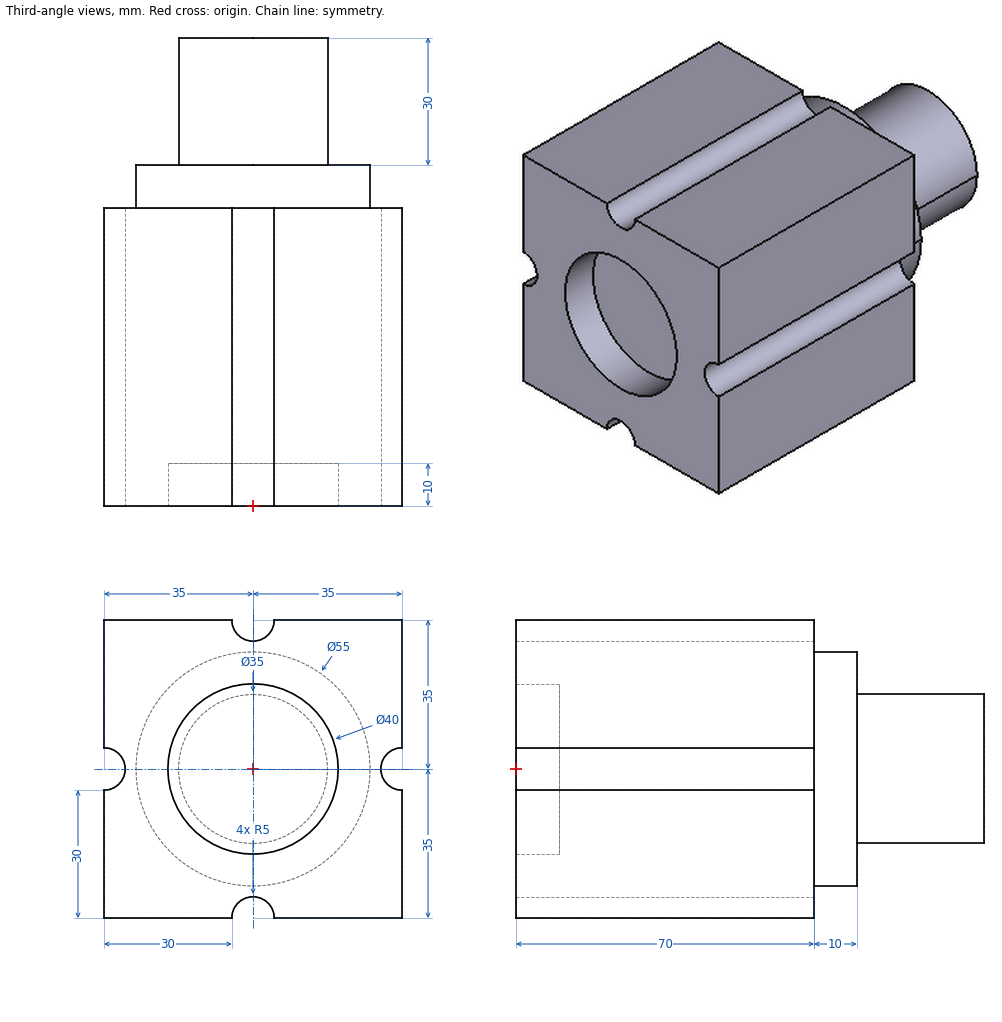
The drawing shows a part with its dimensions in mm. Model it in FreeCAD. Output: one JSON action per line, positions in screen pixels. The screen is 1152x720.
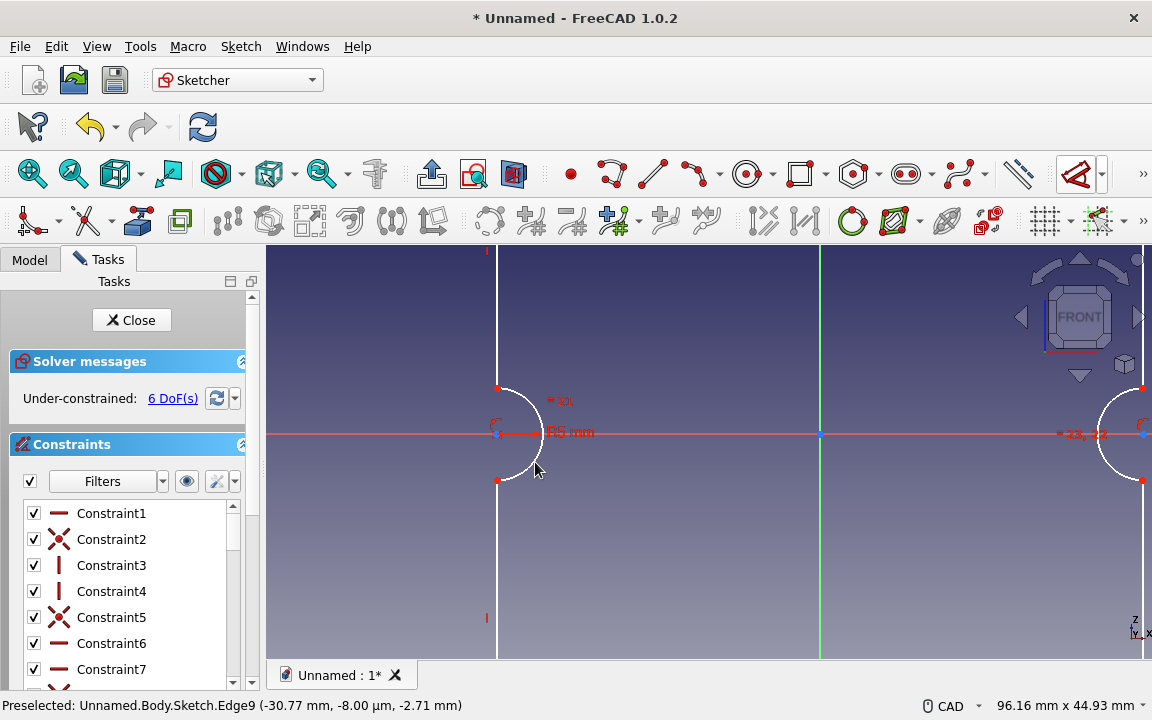
{"action": "scroll", "coordinate": [536, 462], "scroll_direction": "down", "scroll_amount": 5}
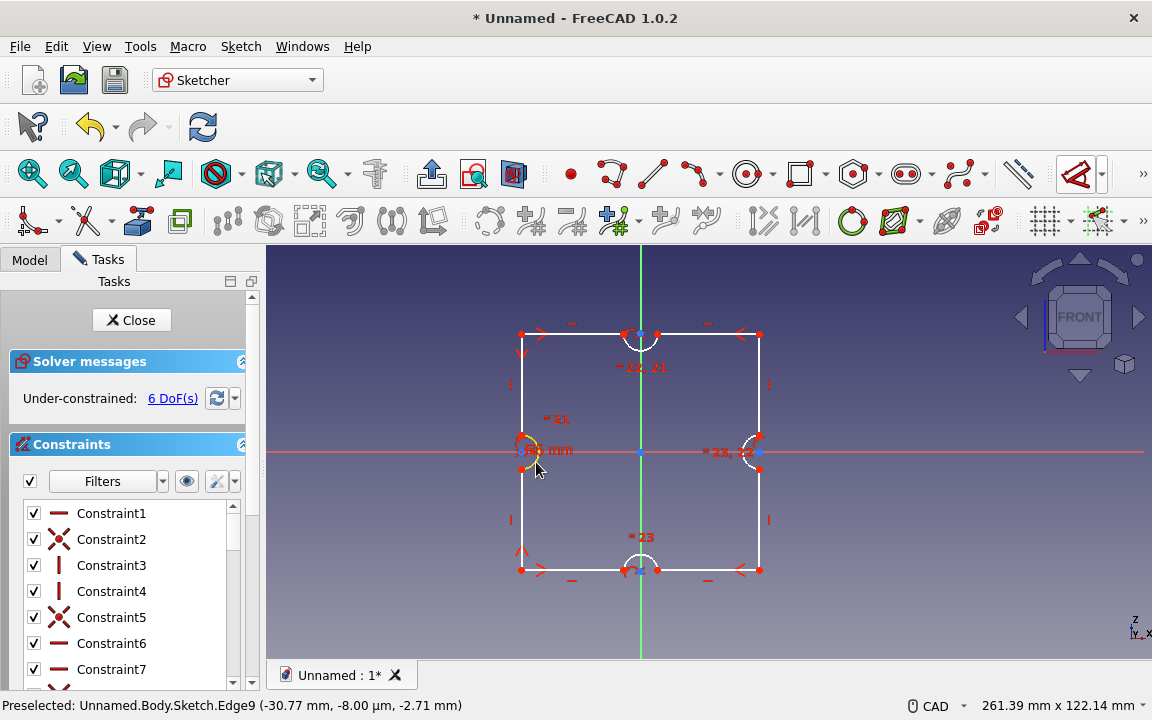
{"action": "left_click", "coordinate": [593, 570]}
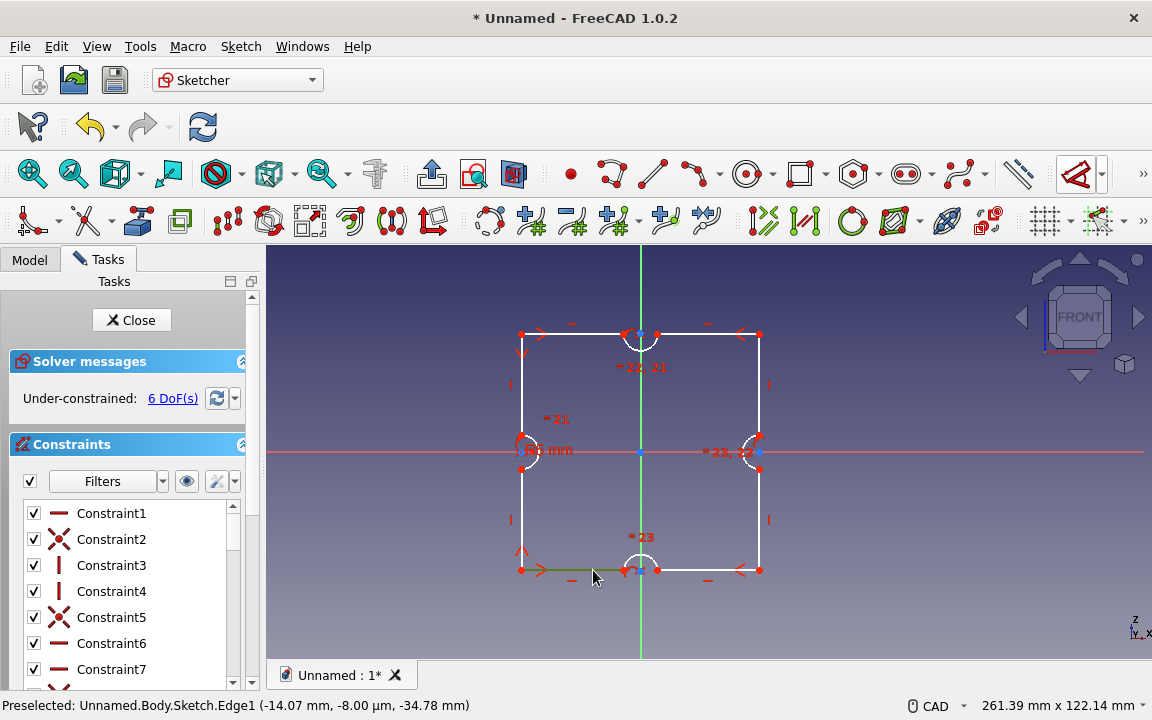
{"action": "key", "text": "l"}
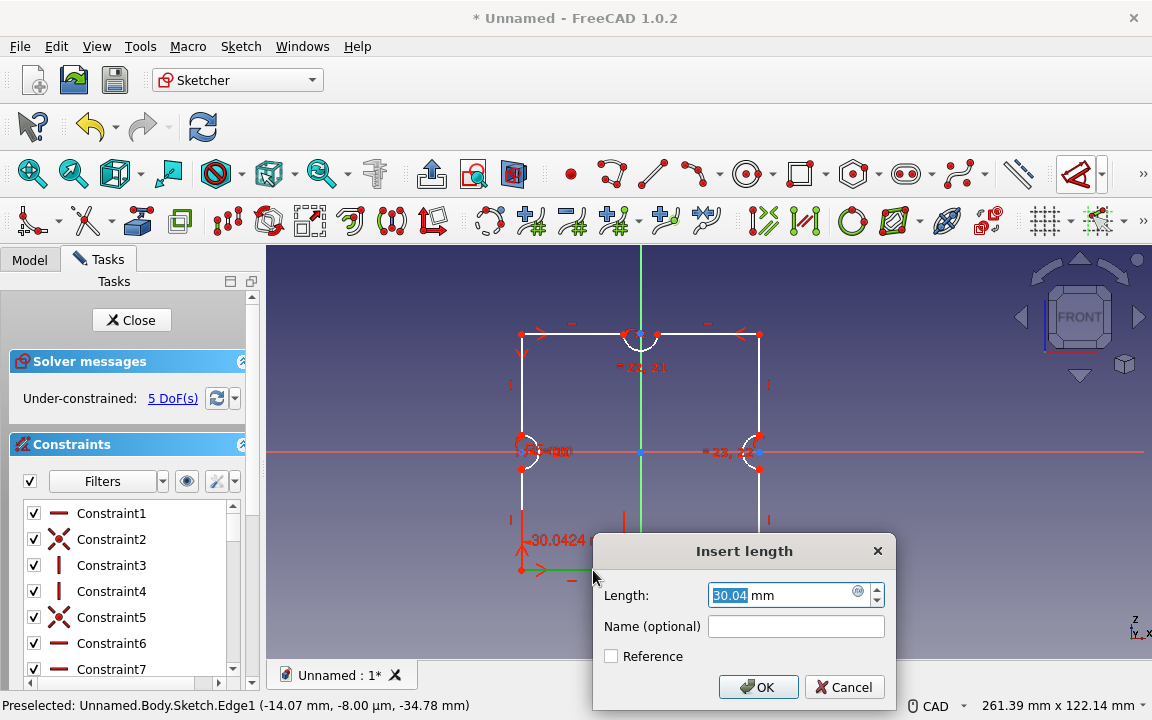
{"action": "type", "text": "30"}
{"action": "key", "text": "Return"}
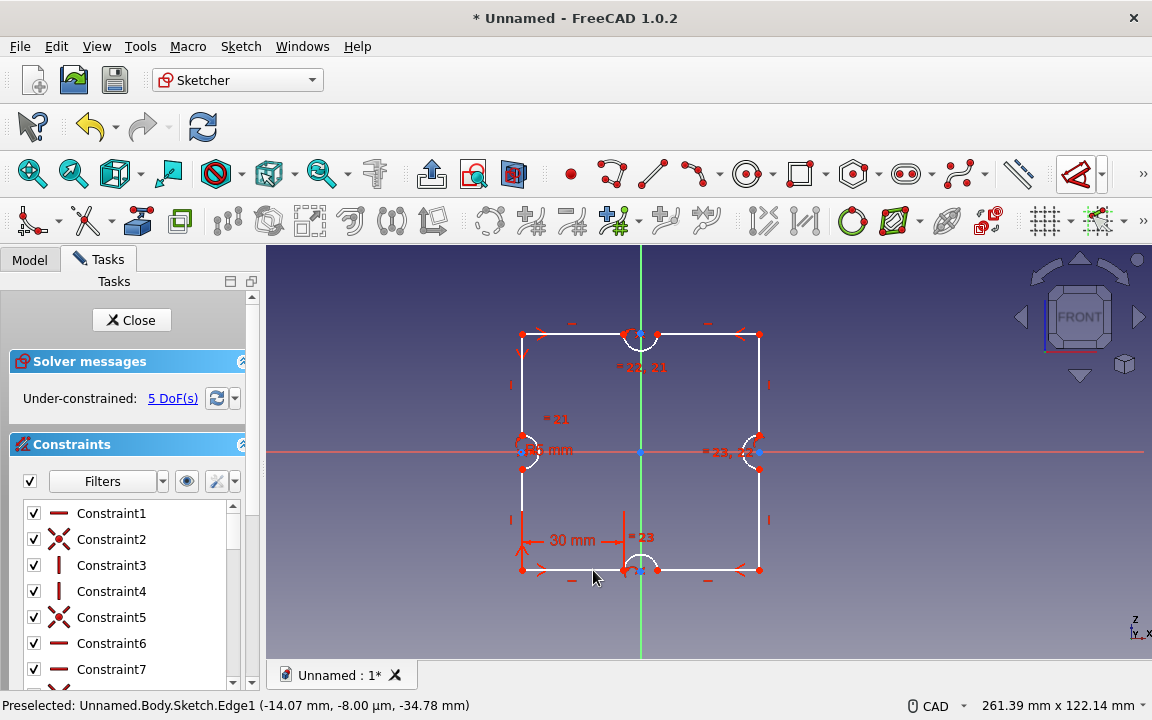
{"action": "left_click", "coordinate": [522, 499]}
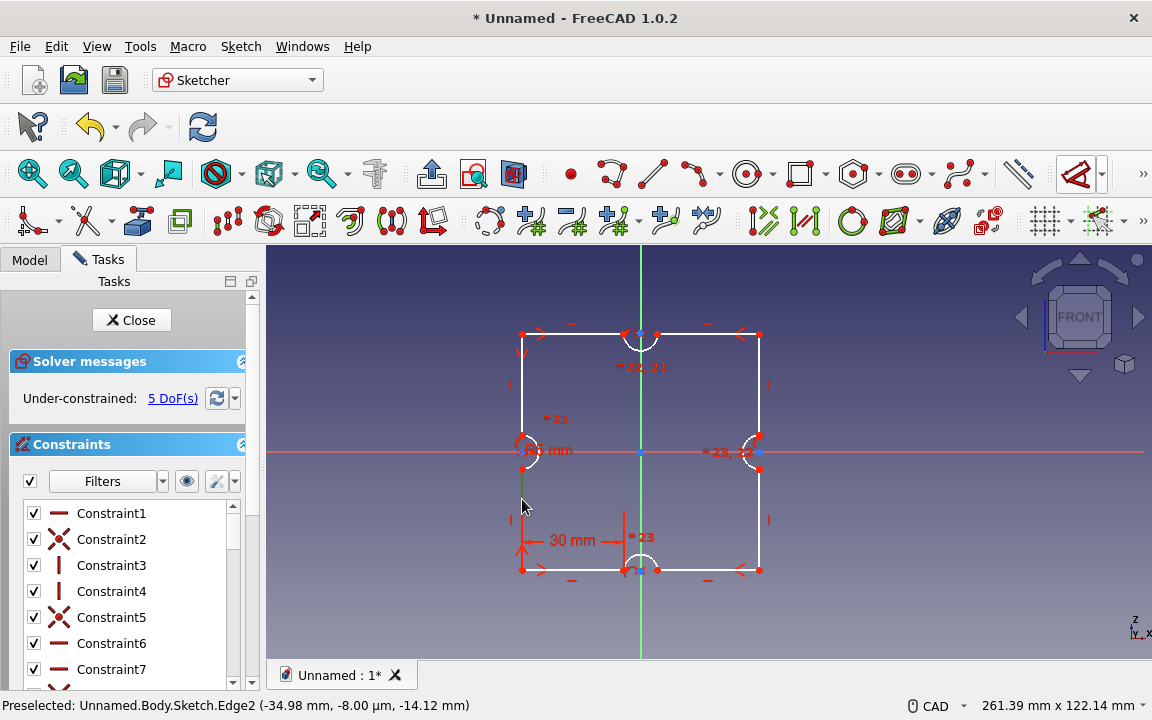
{"action": "left_click", "coordinate": [1102, 174]}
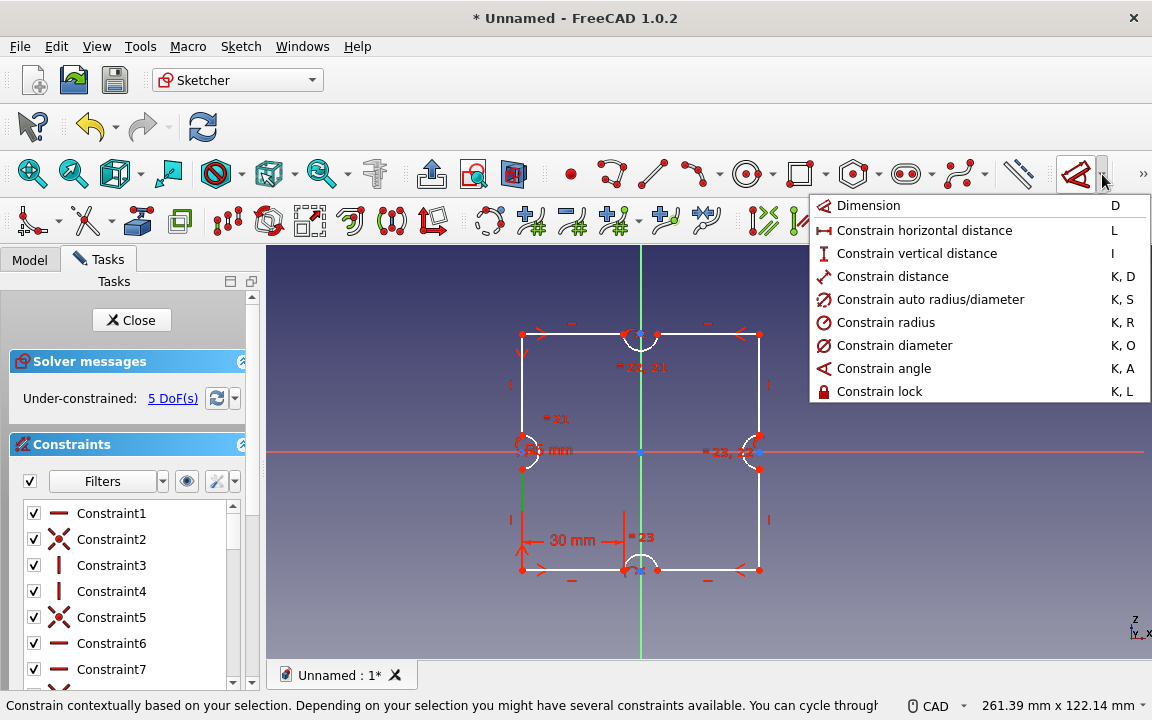
{"action": "left_click", "coordinate": [980, 254]}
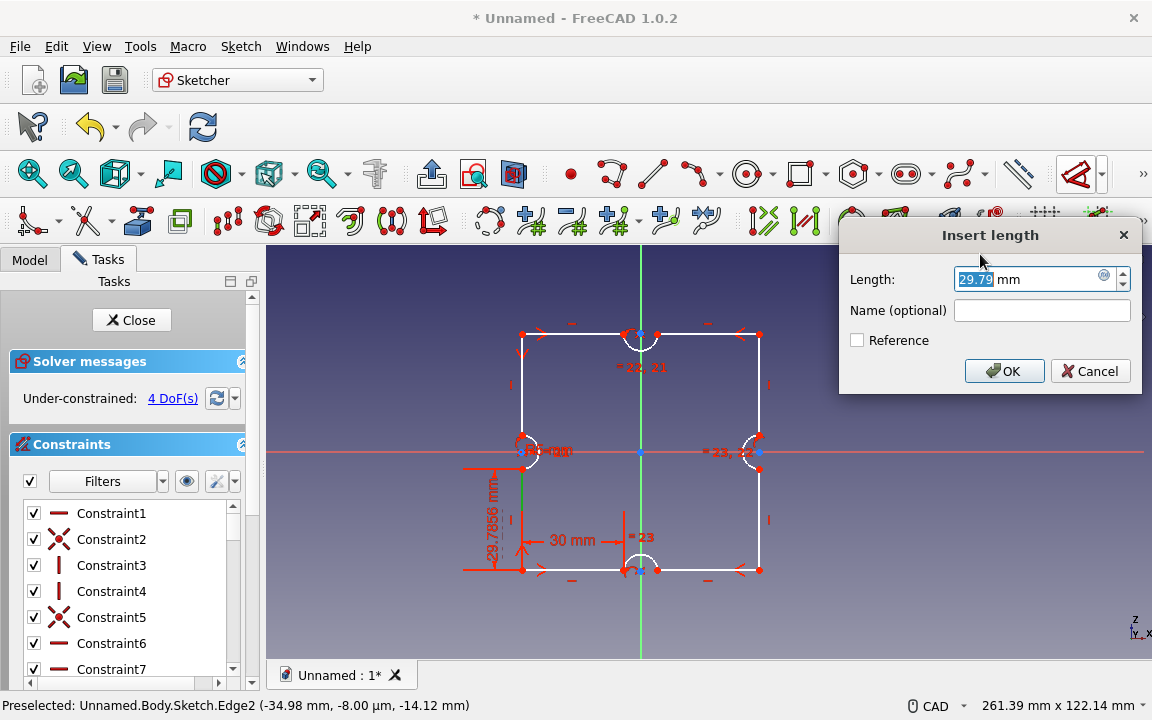
{"action": "type", "text": "30"}
{"action": "key", "text": "Return"}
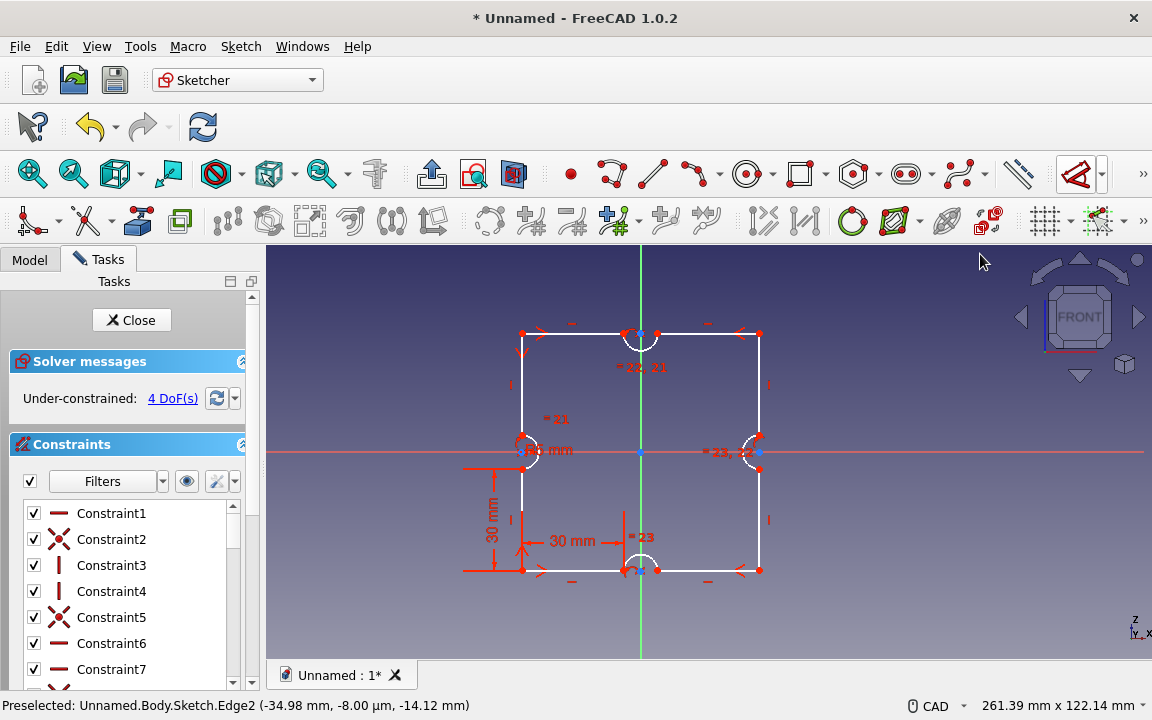
{"action": "left_click", "coordinate": [522, 452]}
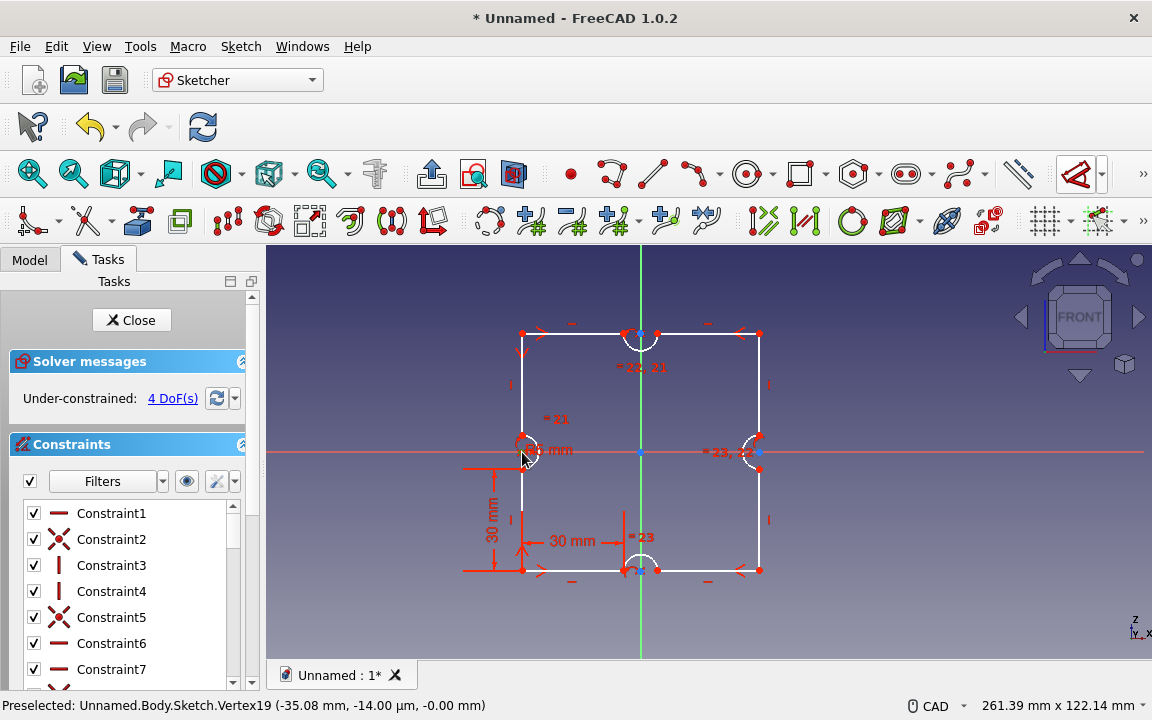
{"action": "key", "text": "l"}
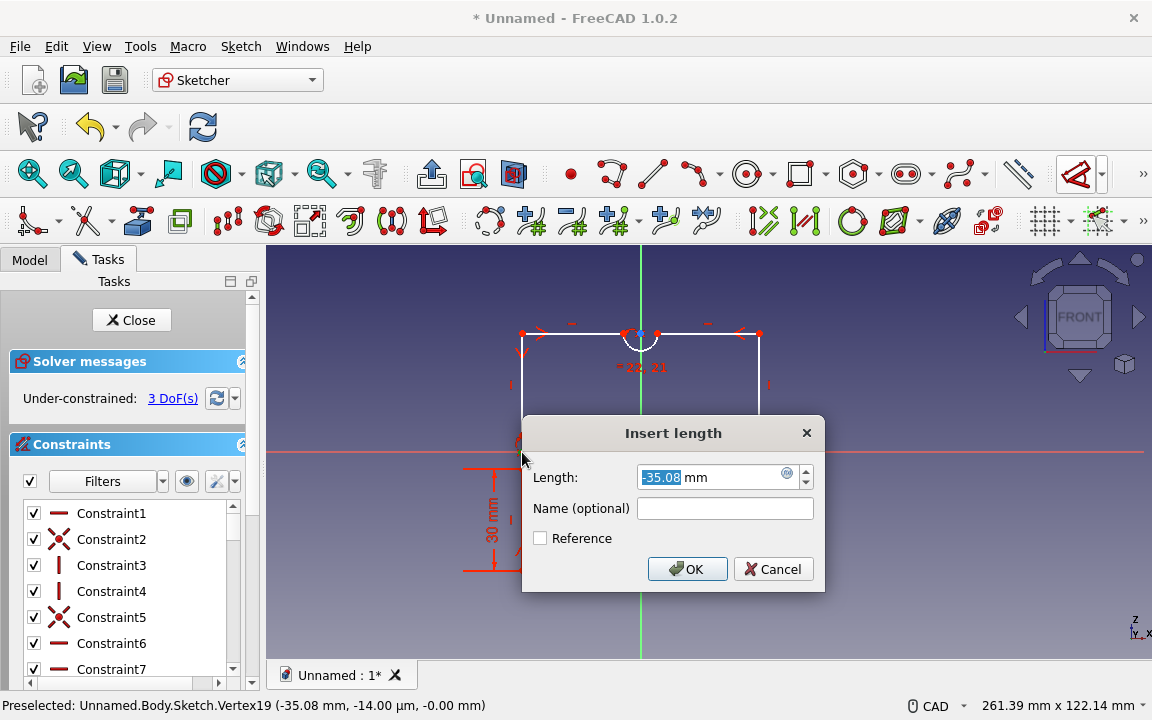
{"action": "type", "text": "-35"}
{"action": "key", "text": "Return"}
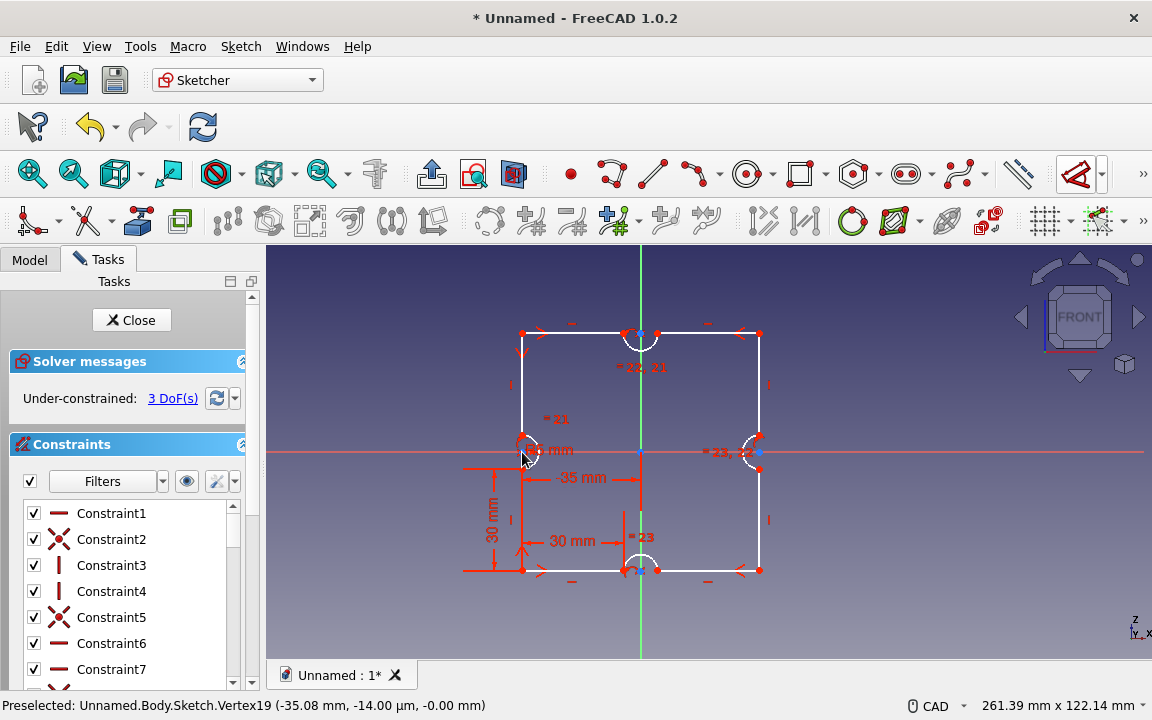
{"action": "left_click", "coordinate": [641, 334]}